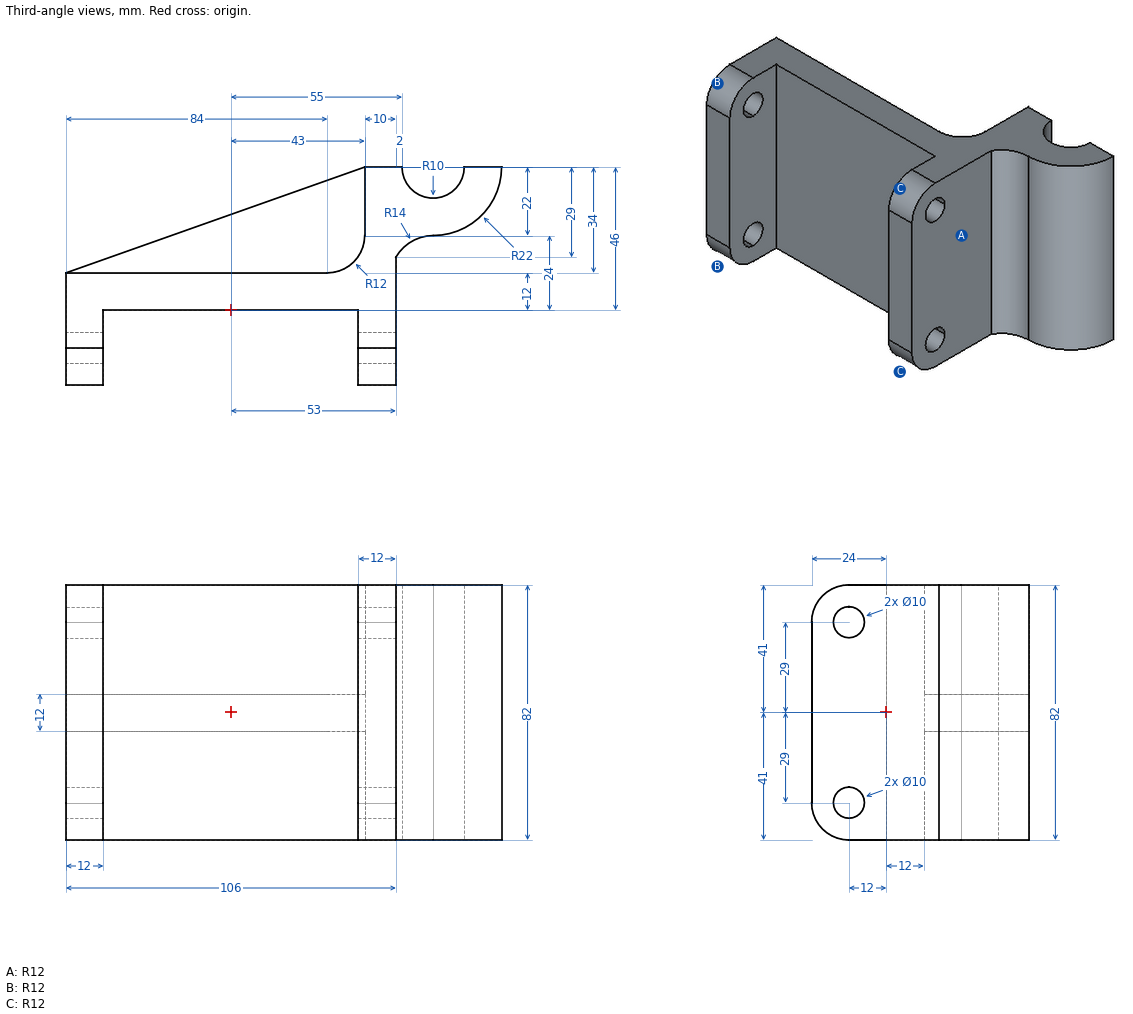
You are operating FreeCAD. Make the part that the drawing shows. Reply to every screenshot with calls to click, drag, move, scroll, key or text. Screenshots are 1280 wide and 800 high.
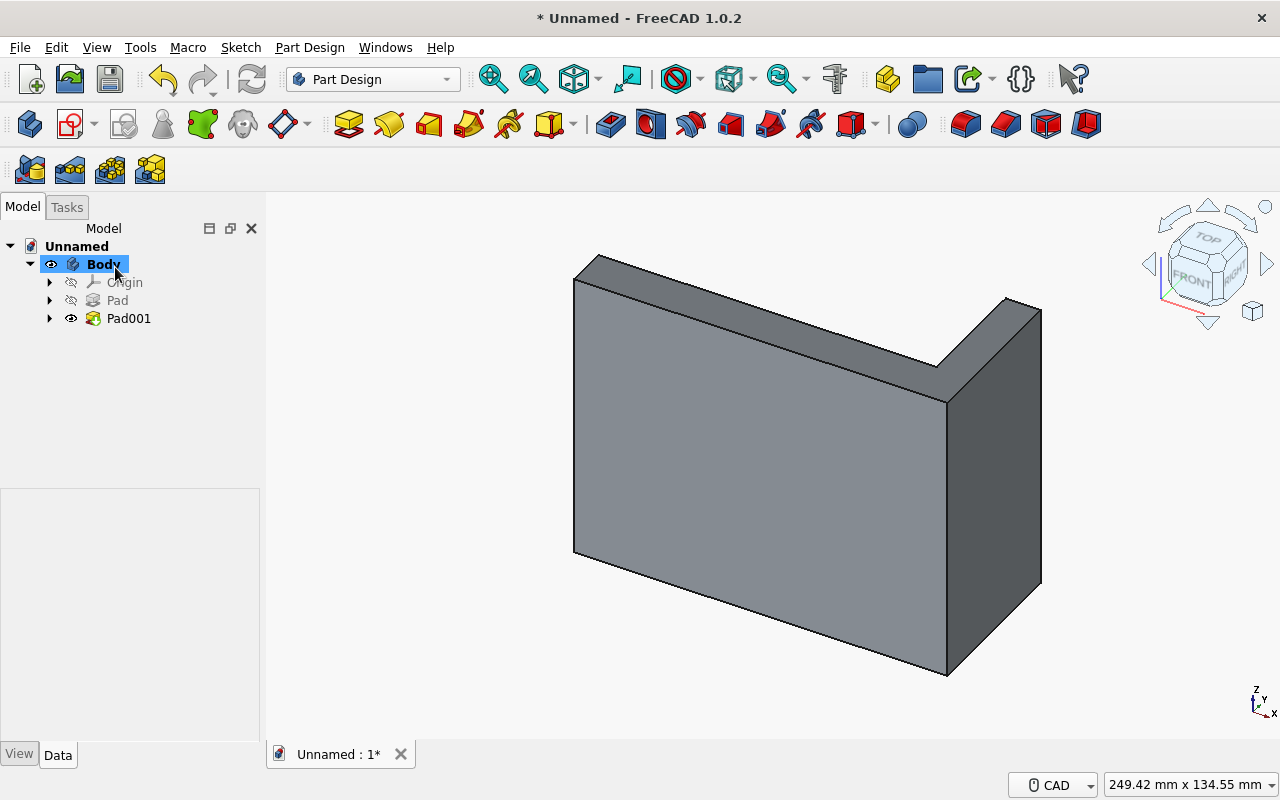
key(v)
key(f)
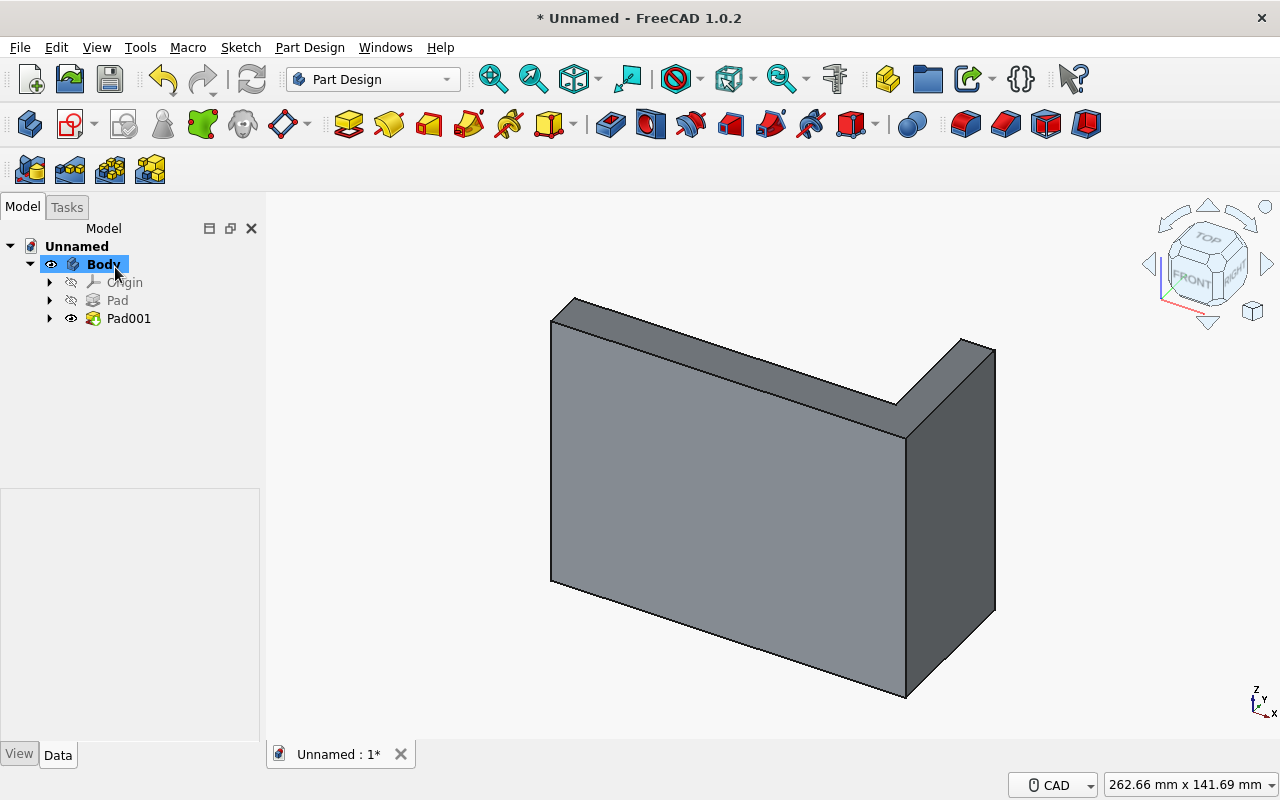
key(0)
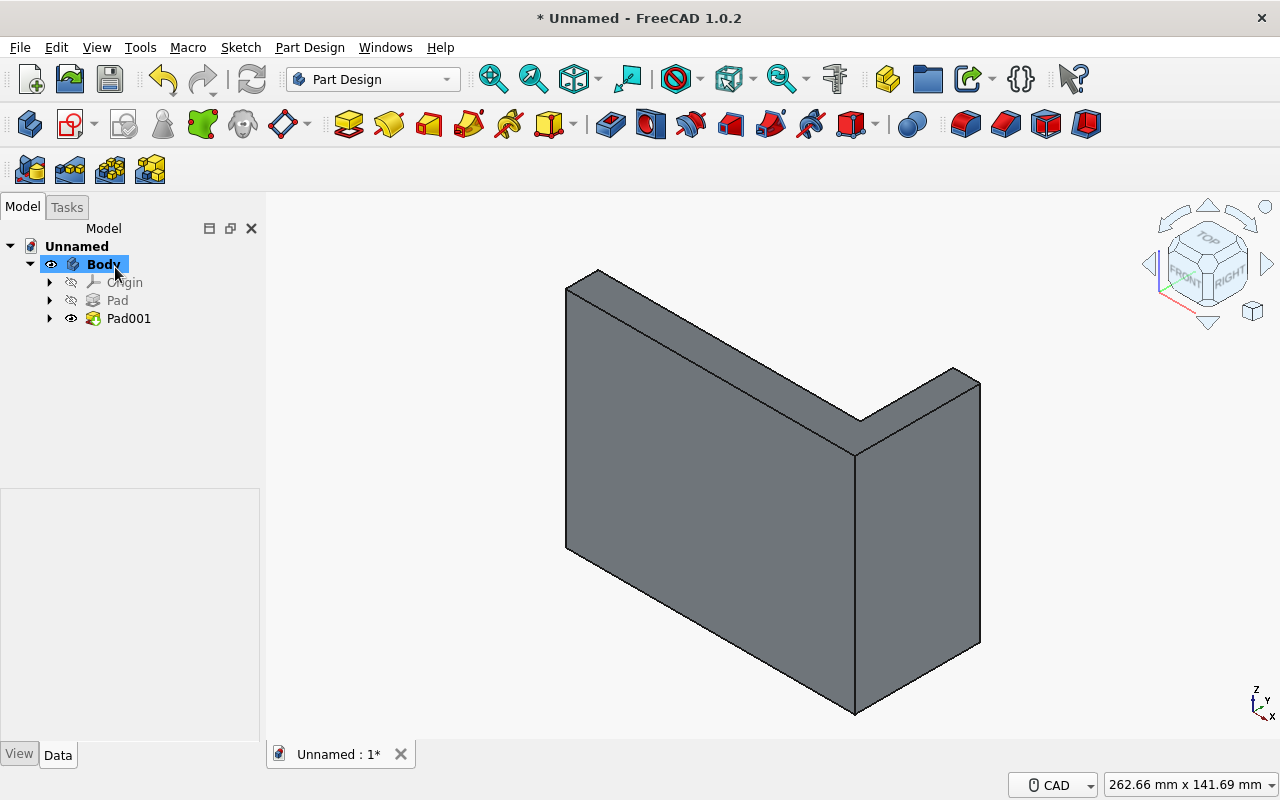
key(2)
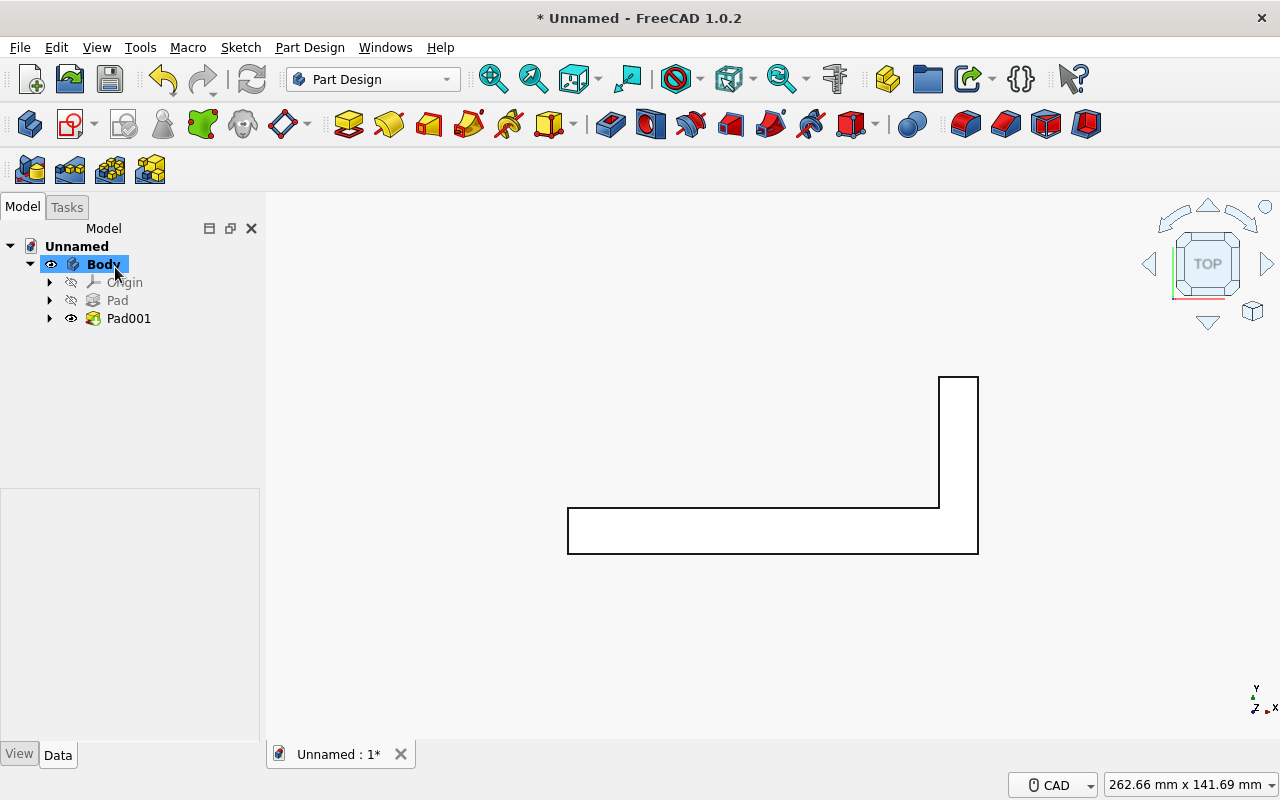
key(v)
key(f)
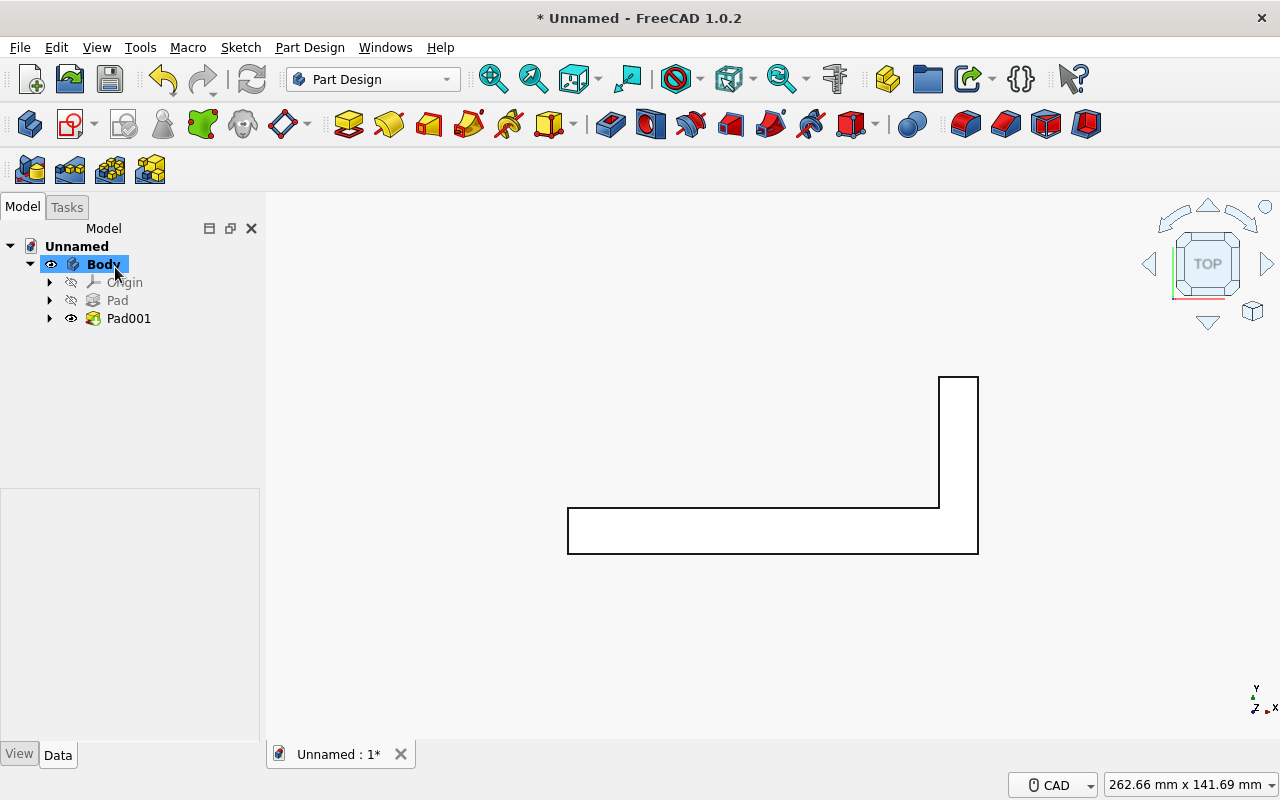
key(1)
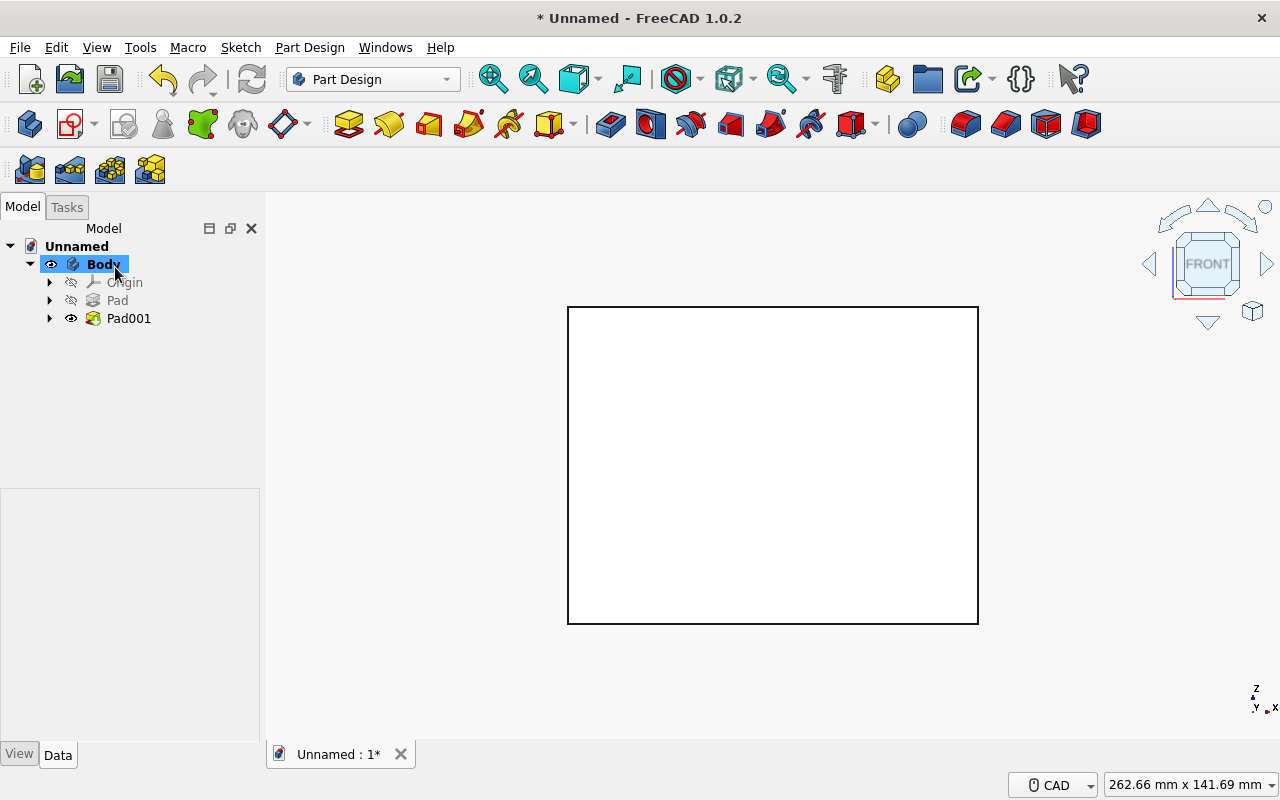
key(3)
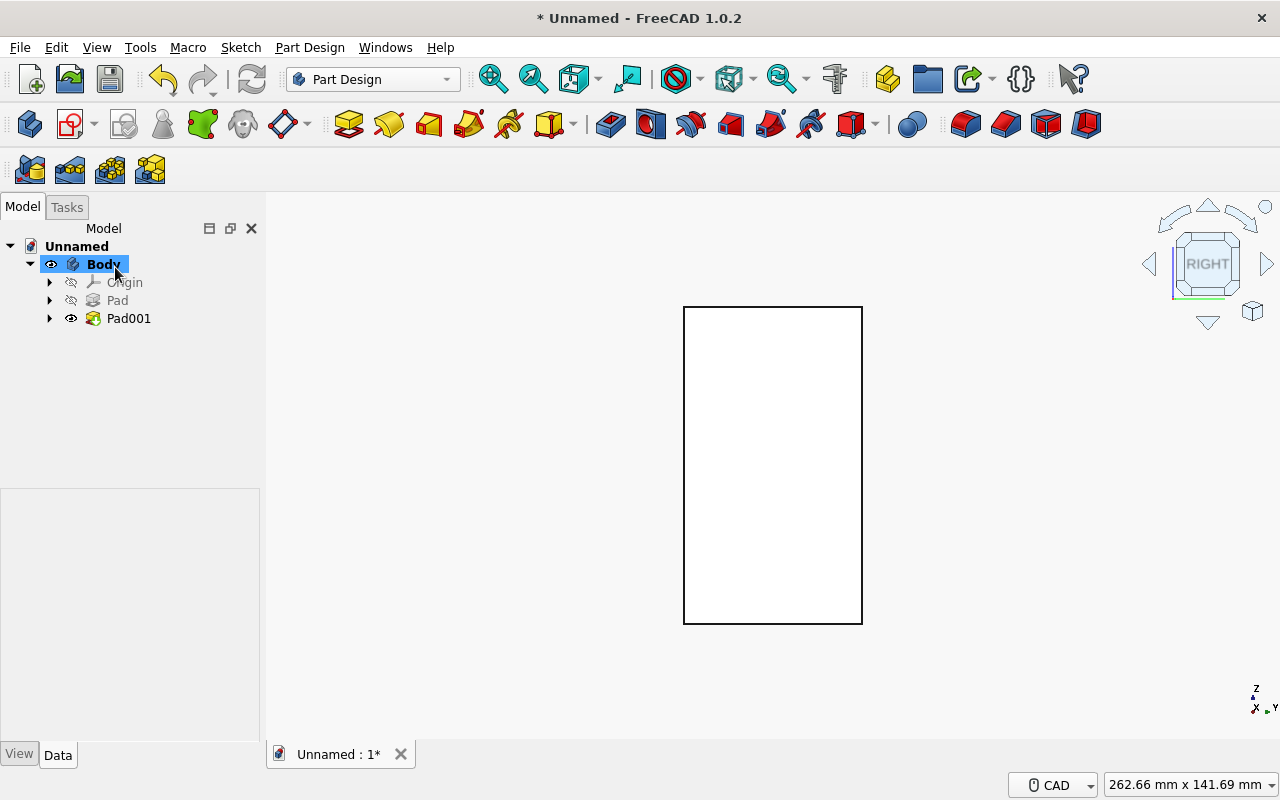
key(5)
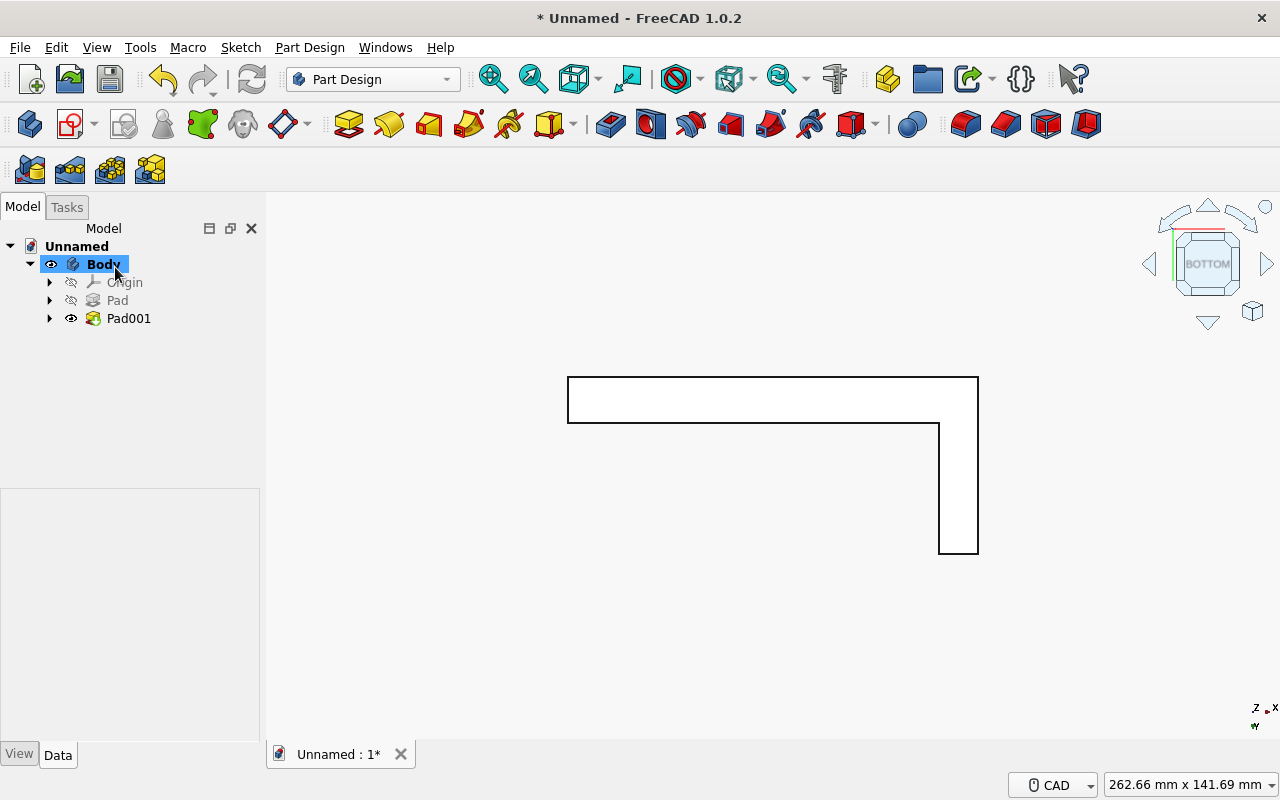
click(494, 80)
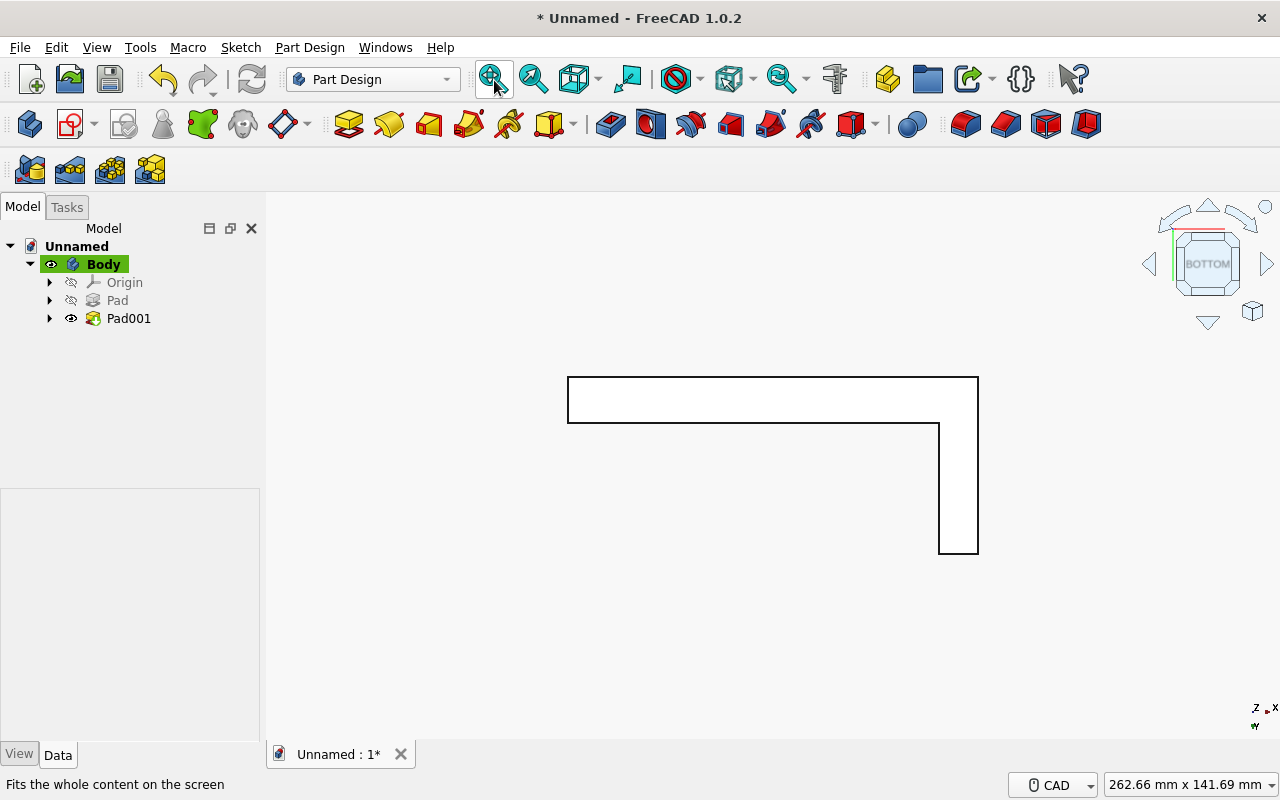
key(4)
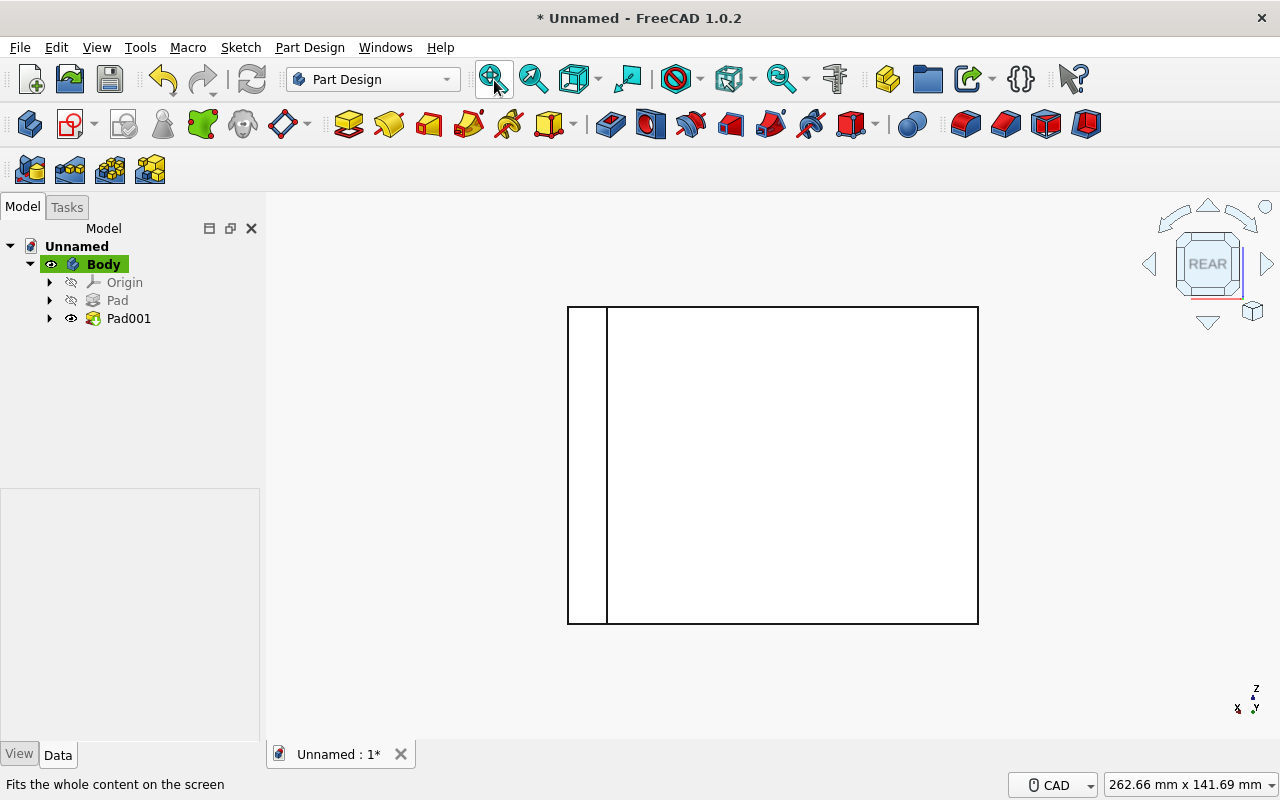
key(6)